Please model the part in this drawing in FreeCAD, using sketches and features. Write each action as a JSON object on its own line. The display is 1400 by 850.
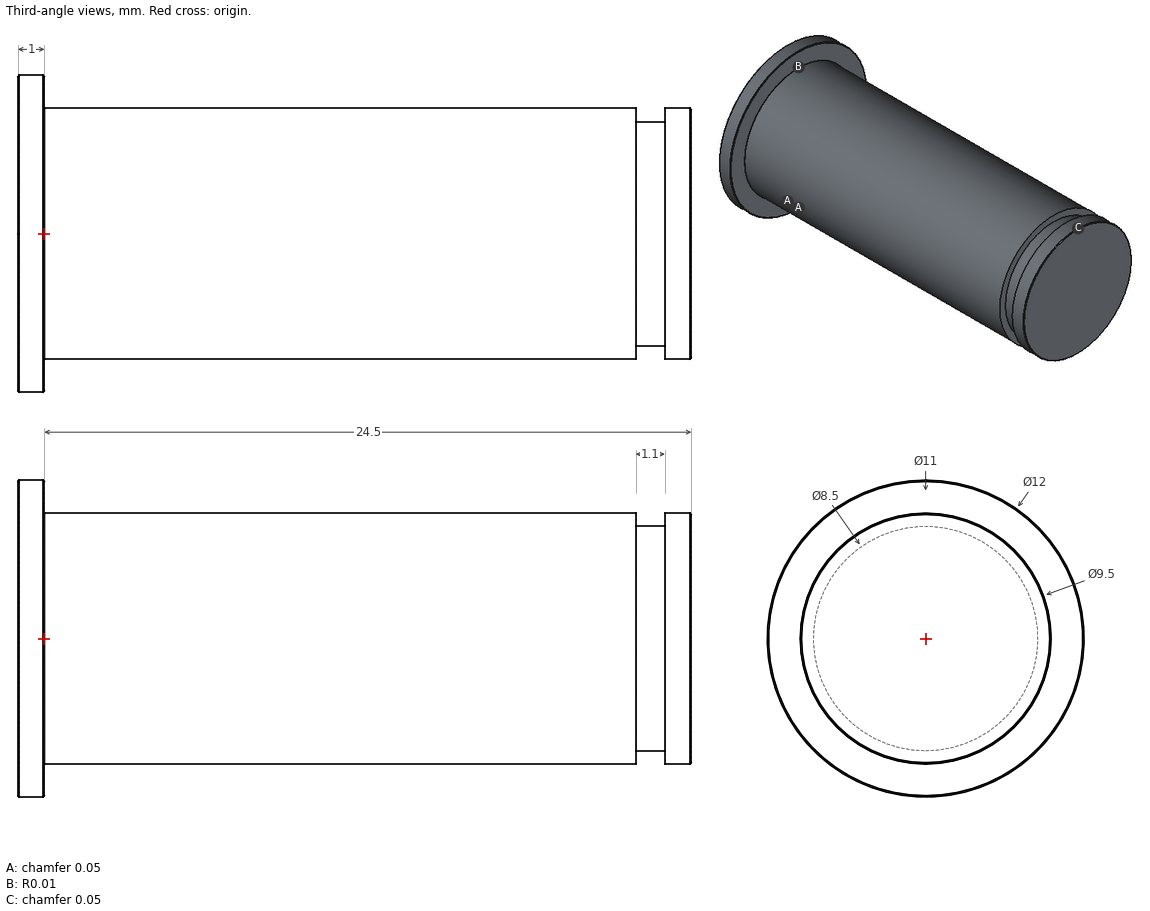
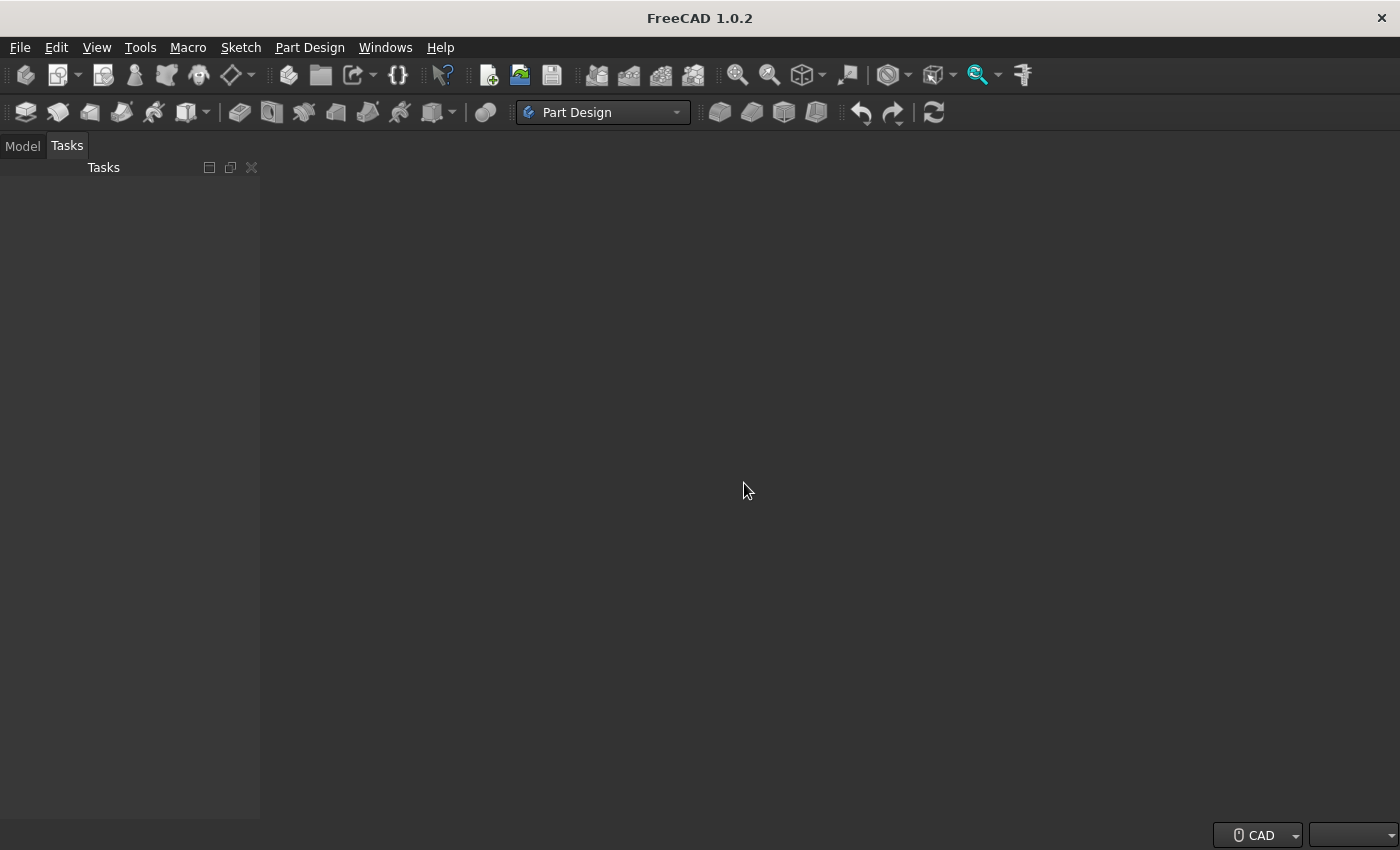
{"action": "key", "text": "ctrl+n"}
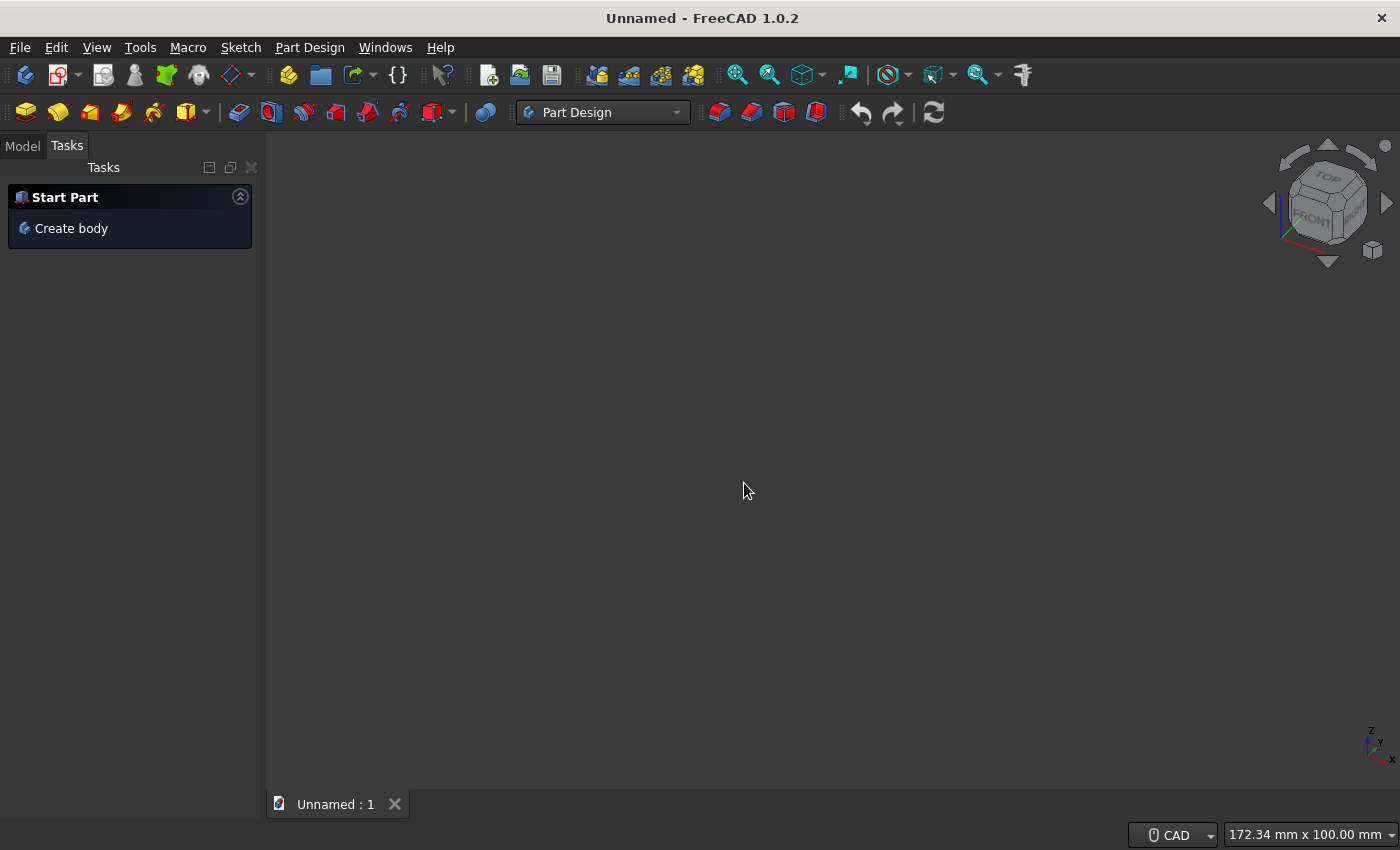
{"action": "left_click", "coordinate": [58, 76]}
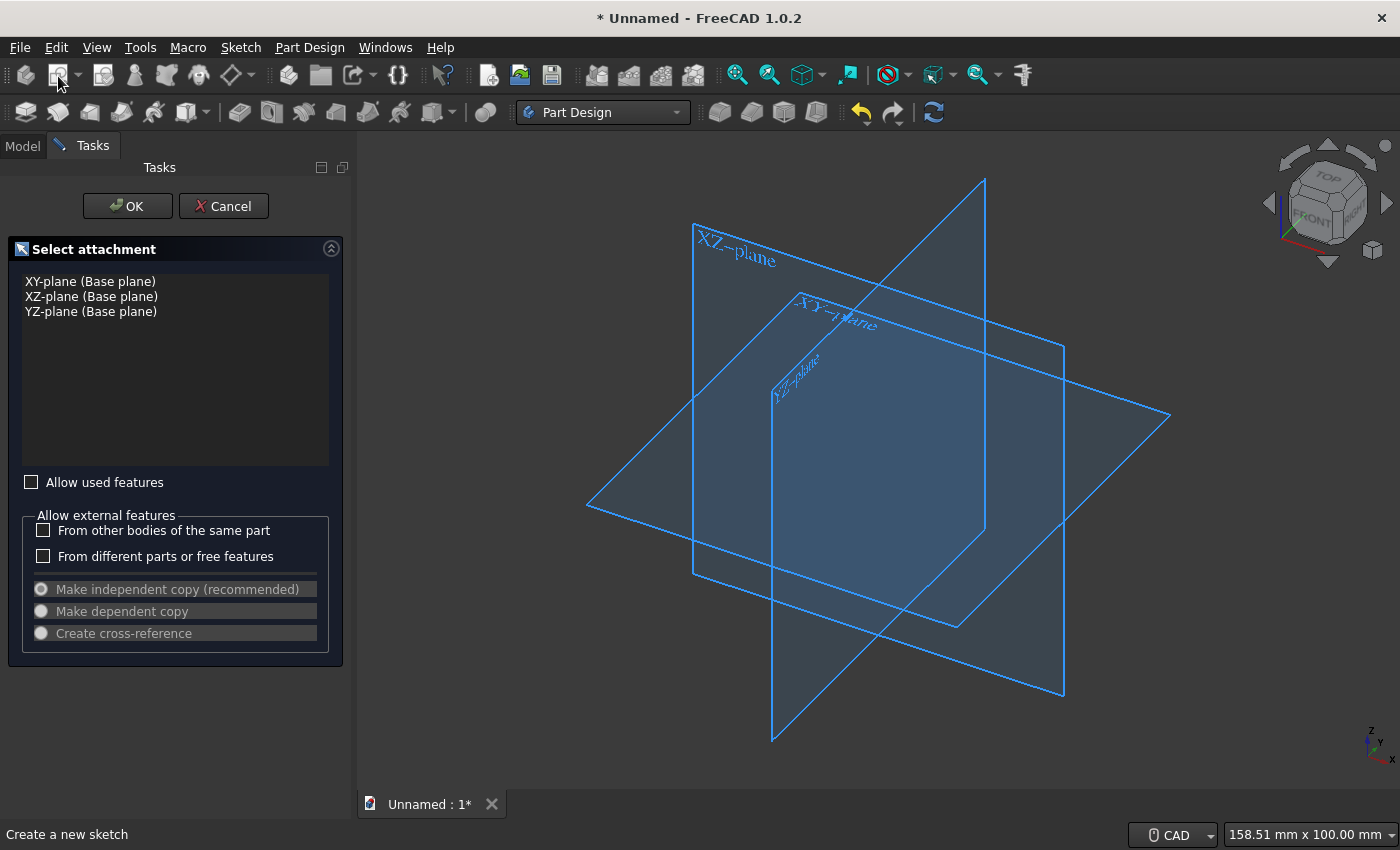
{"action": "left_click", "coordinate": [82, 312]}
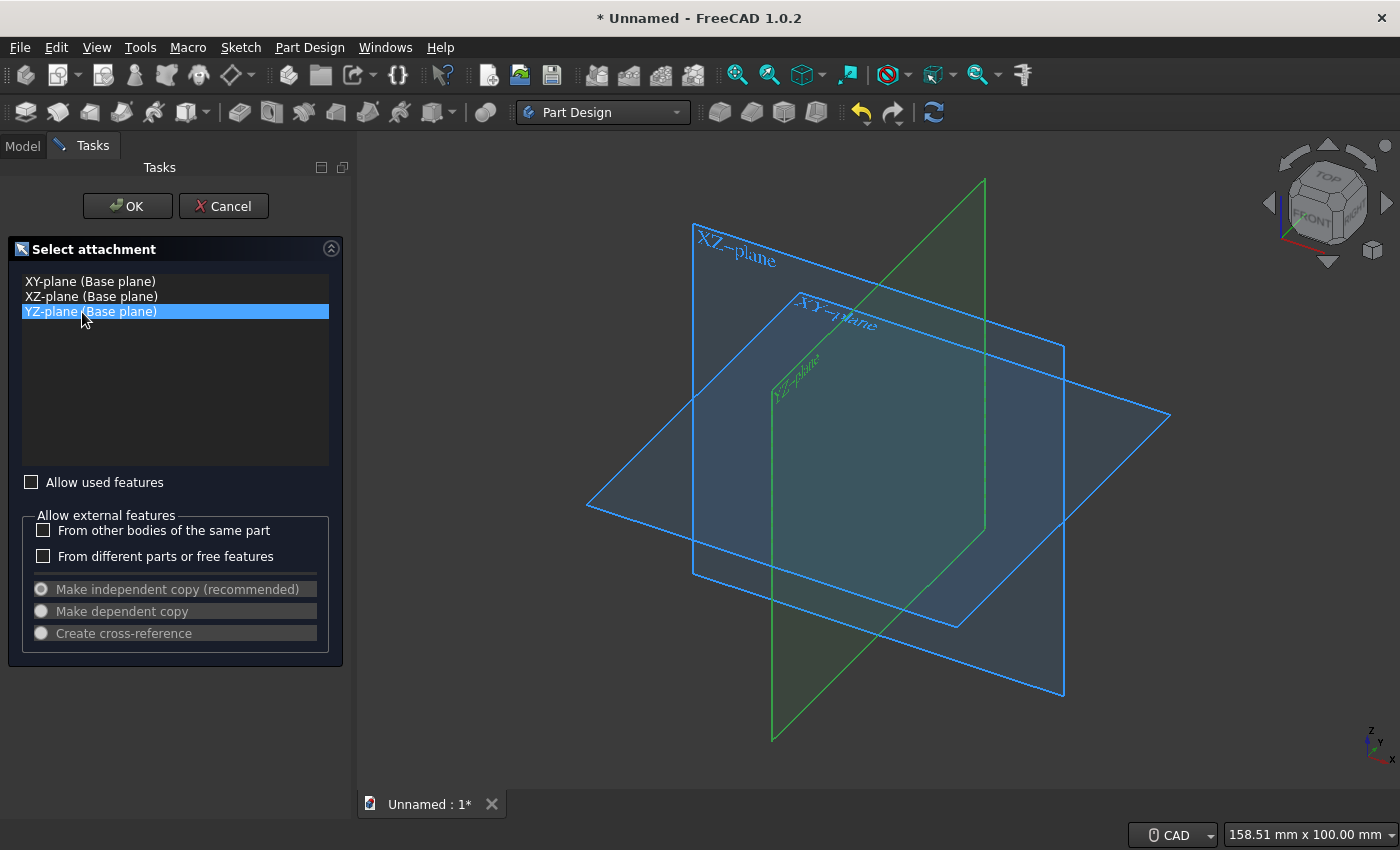
{"action": "left_click", "coordinate": [128, 206]}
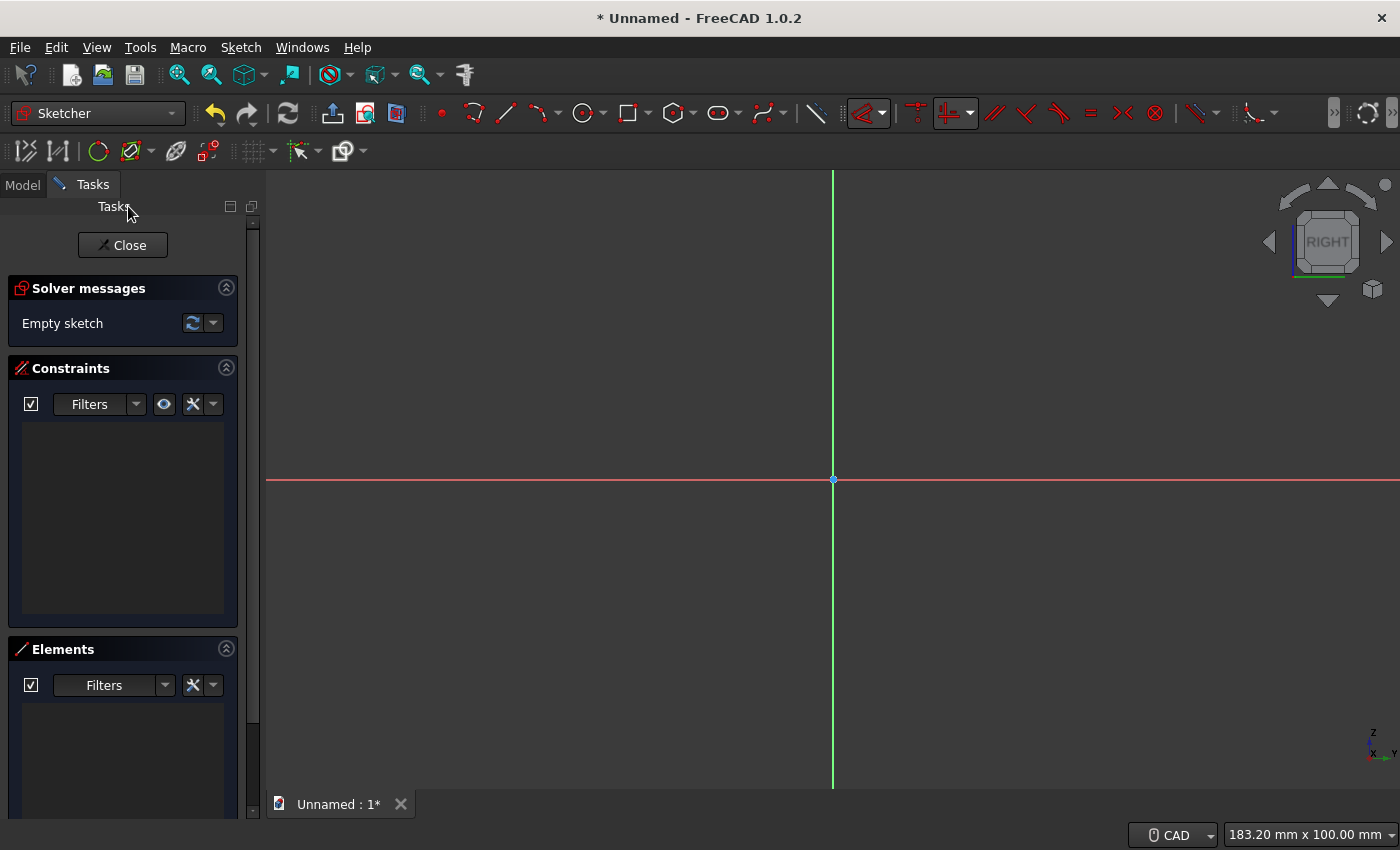
{"action": "scroll", "coordinate": [844, 480], "scroll_direction": "up", "scroll_amount": 10}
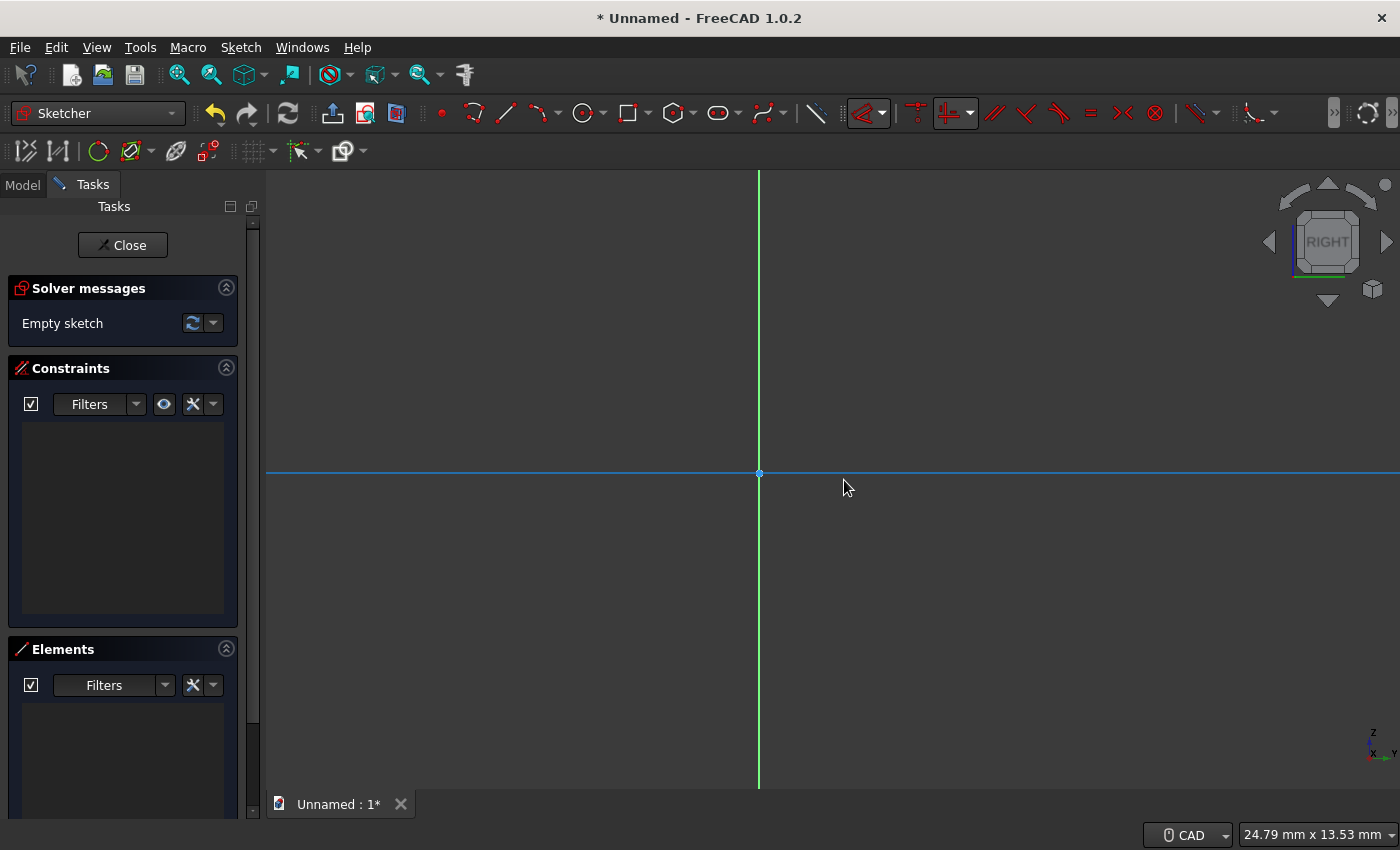
{"action": "key", "text": "g c"}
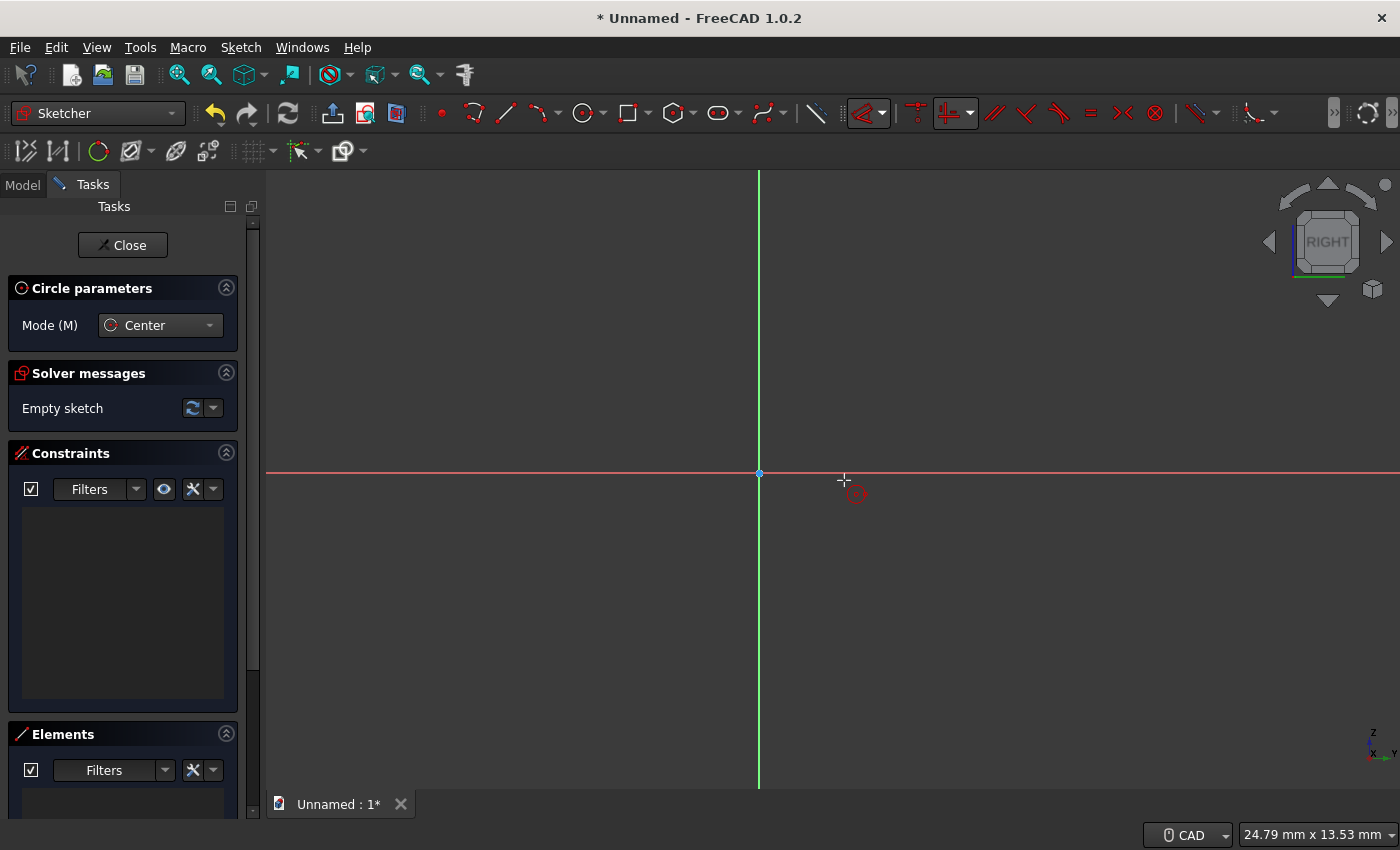
{"action": "left_click", "coordinate": [759, 473]}
{"action": "left_click", "coordinate": [913, 319]}
{"action": "key", "text": "Escape"}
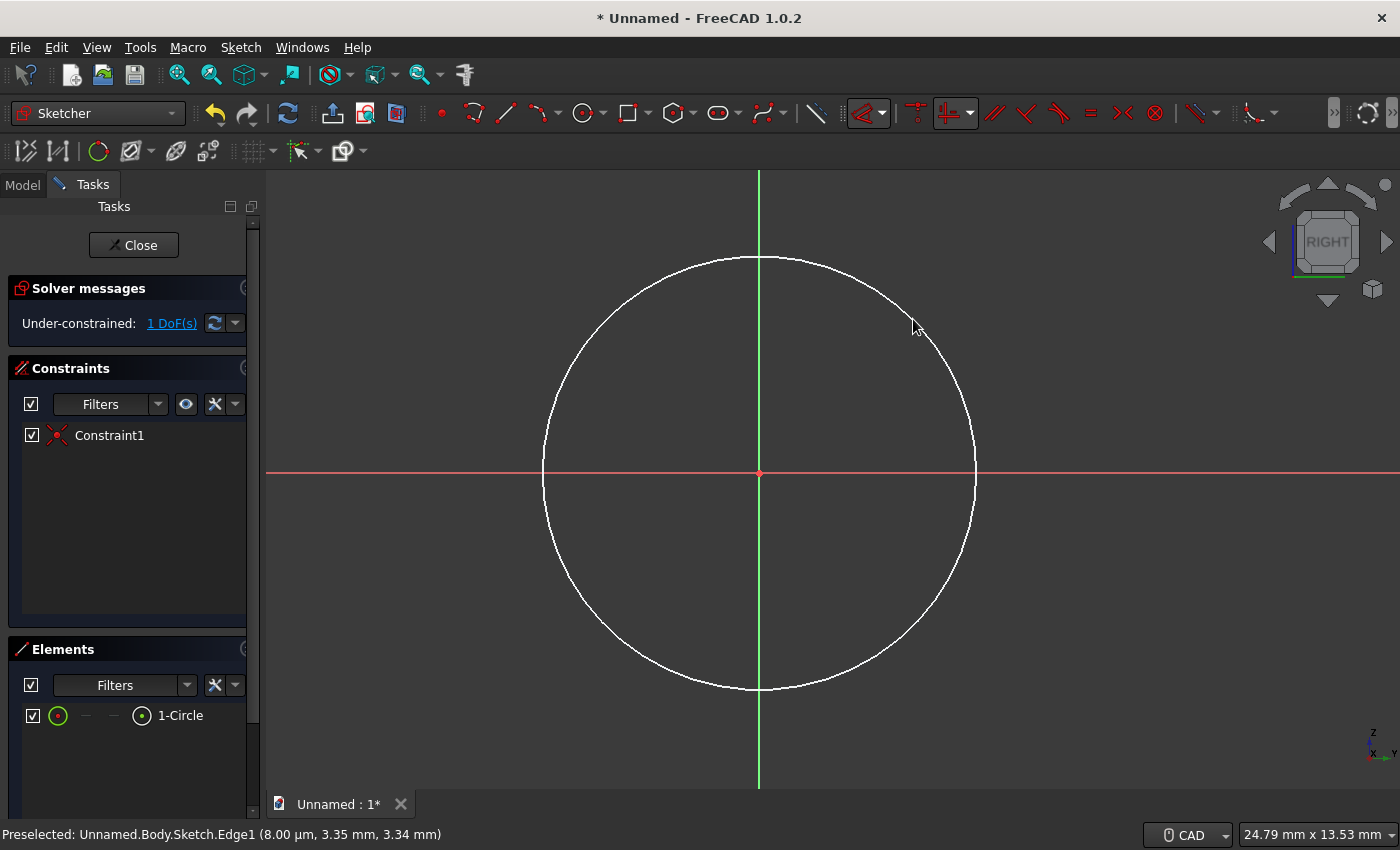
{"action": "key", "text": "d"}